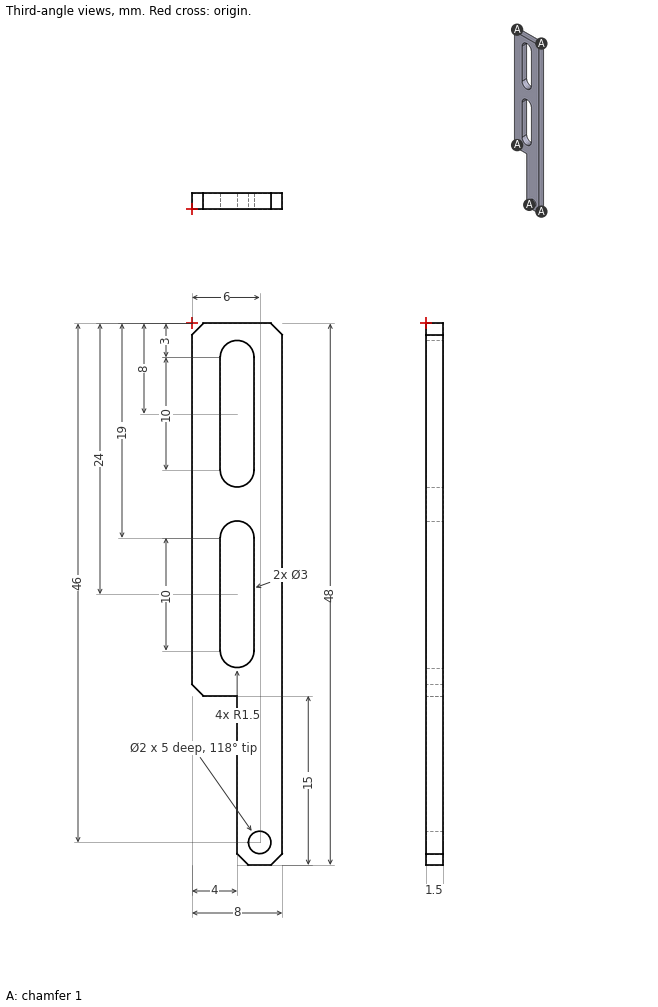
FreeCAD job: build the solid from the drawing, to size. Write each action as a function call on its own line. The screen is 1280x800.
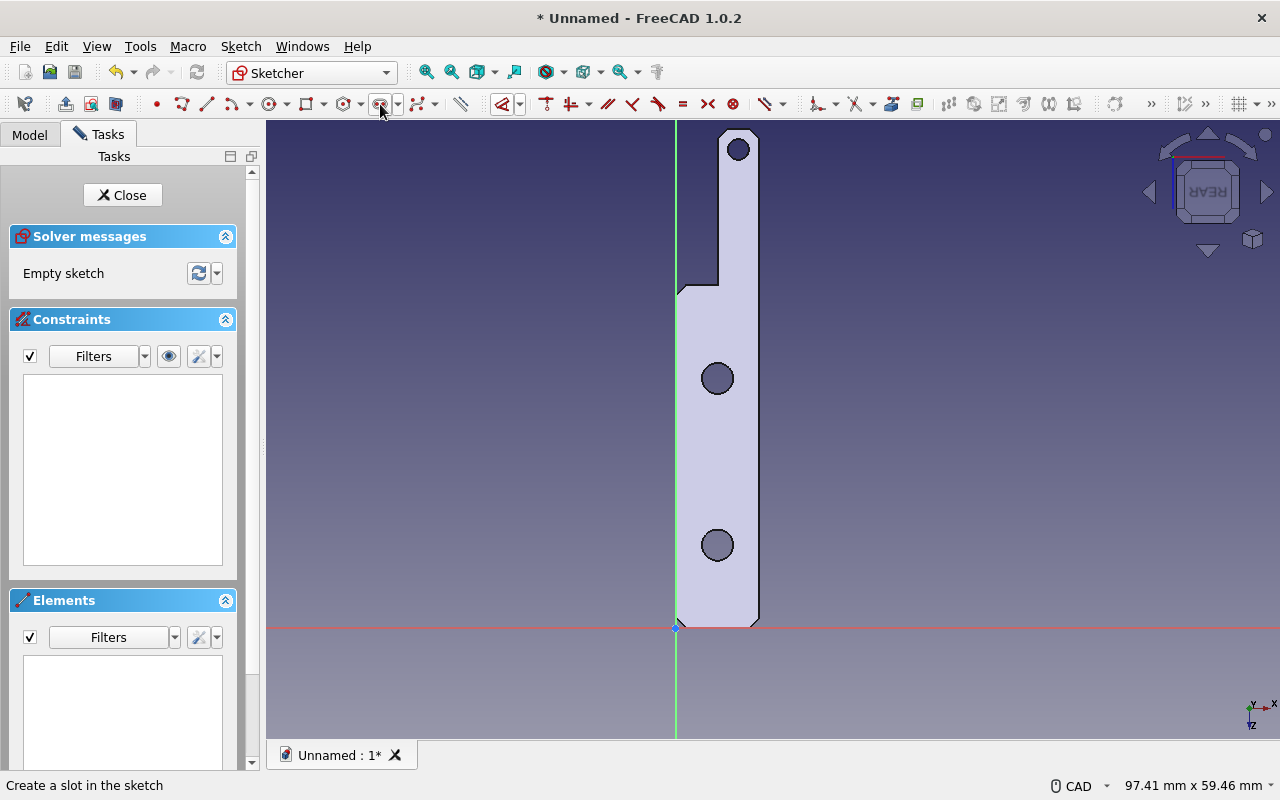
scroll(718, 431, up, 2)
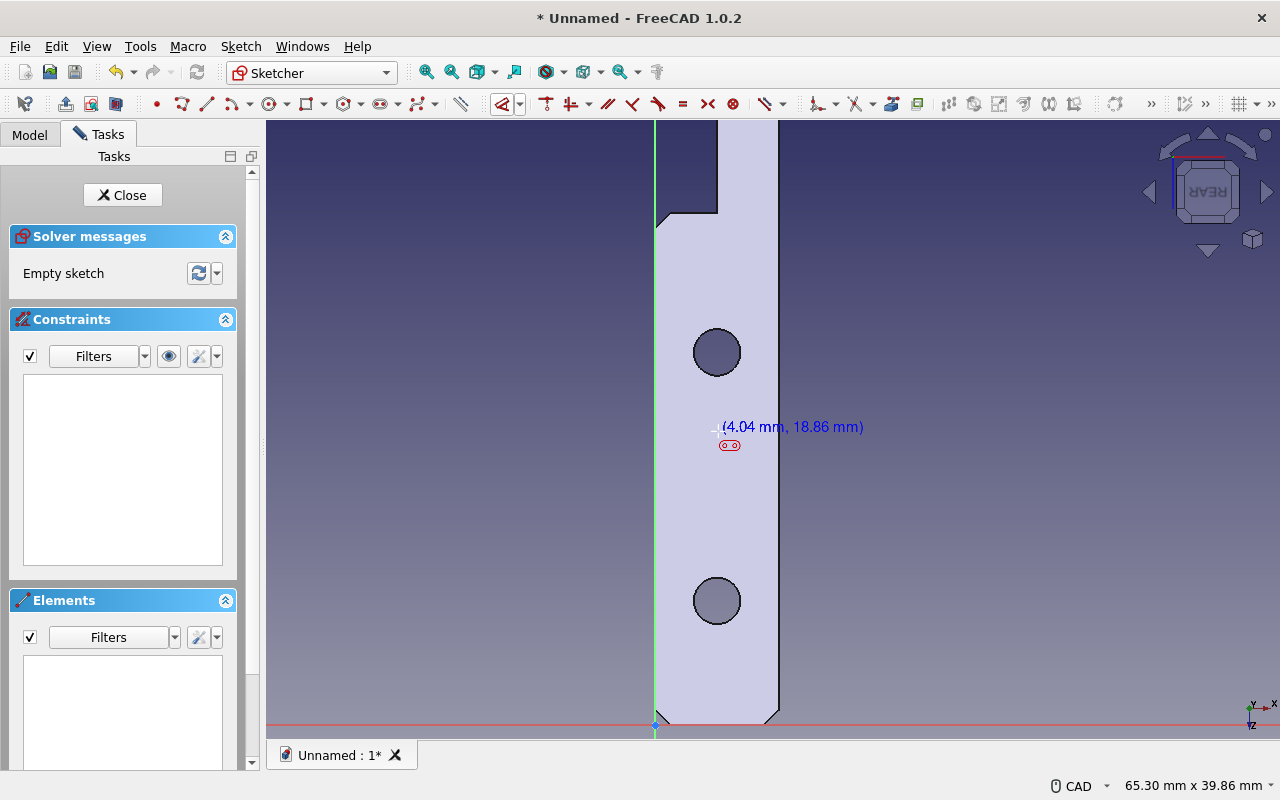
click(717, 430)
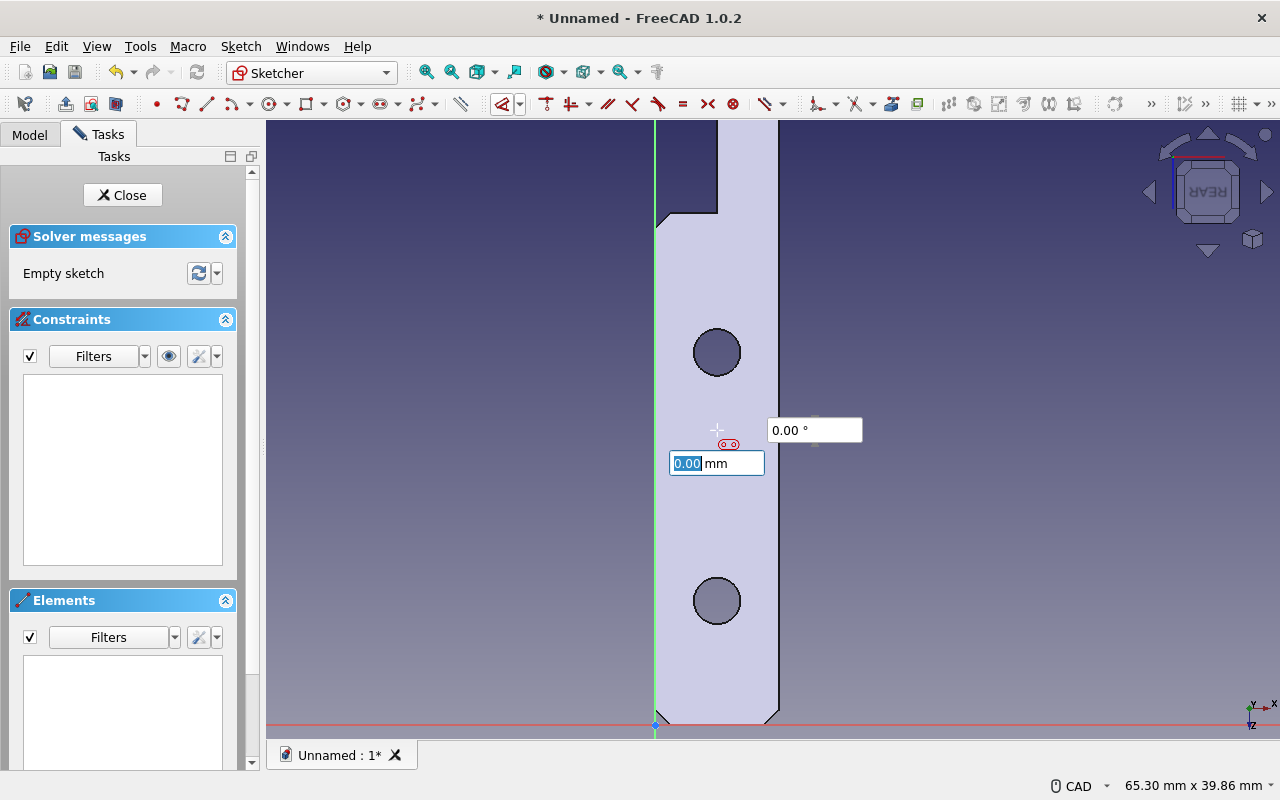
click(717, 275)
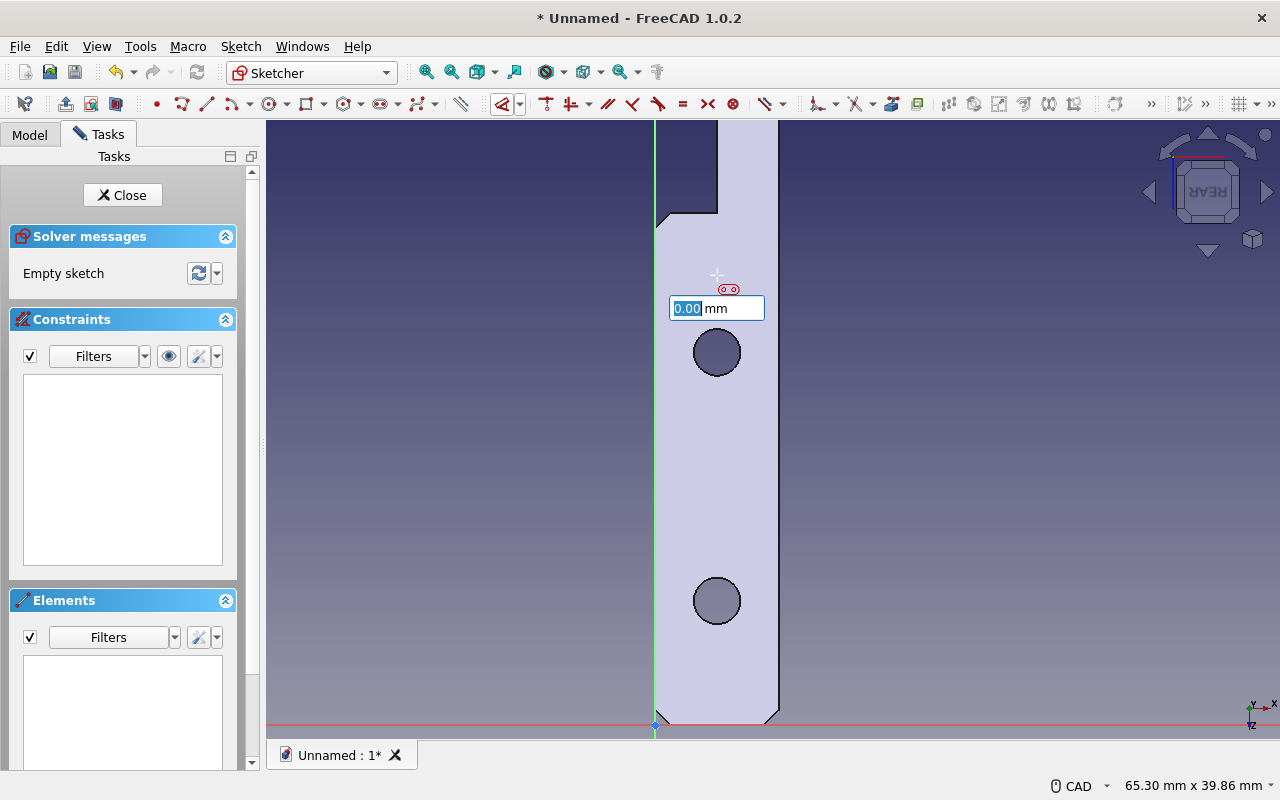
click(740, 352)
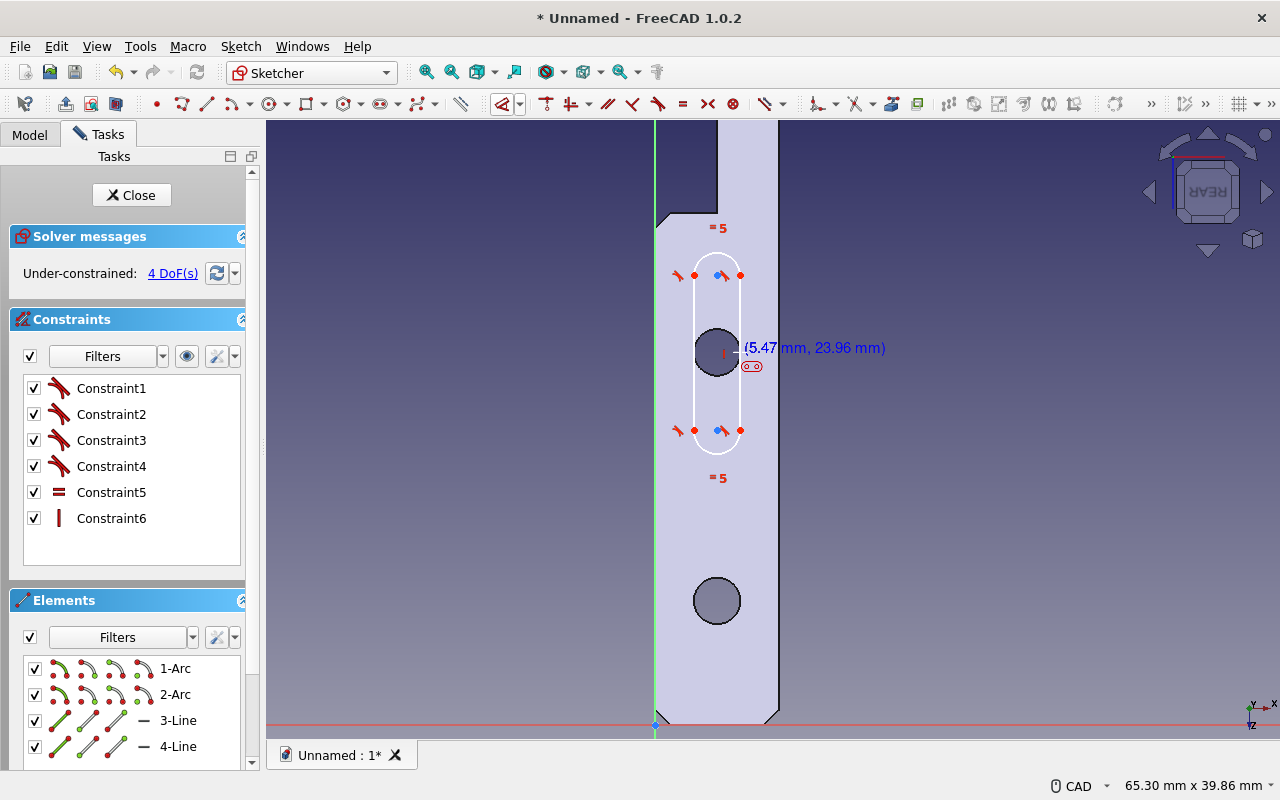
click(717, 679)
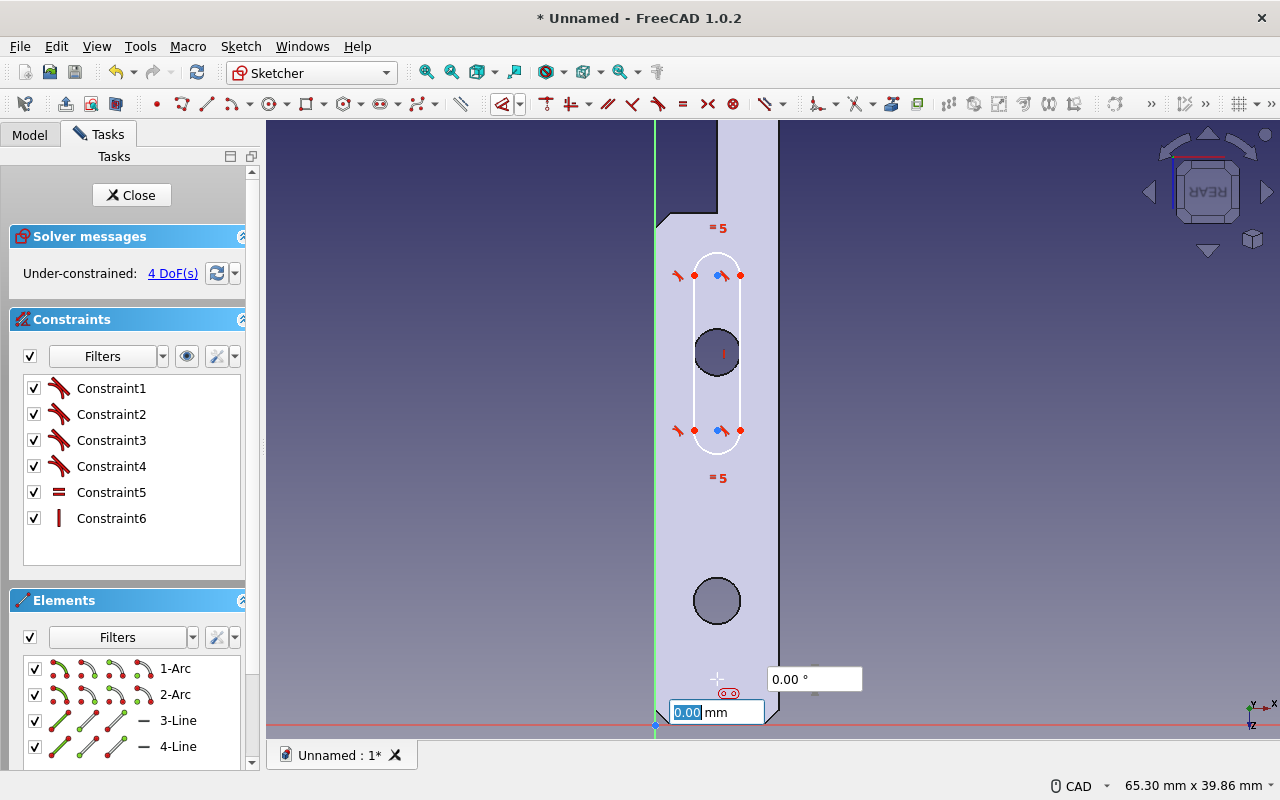
click(717, 523)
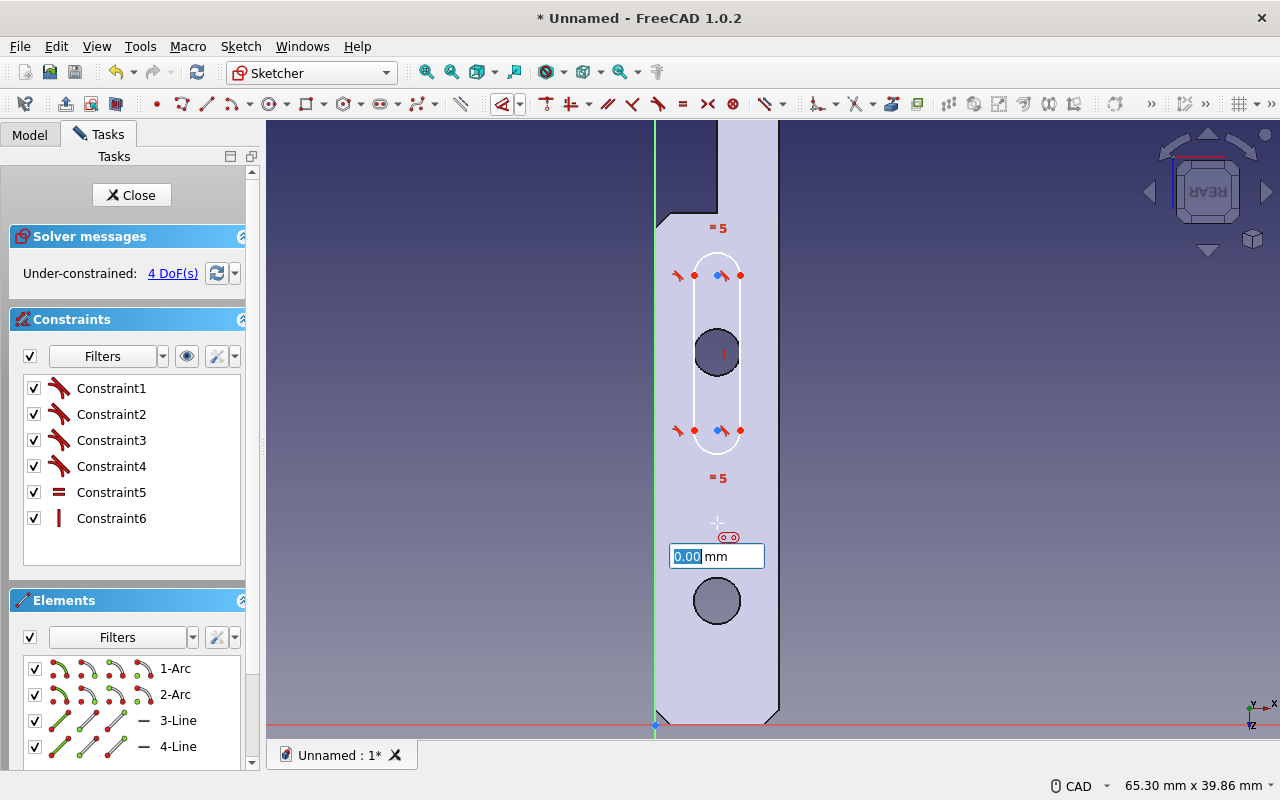
click(694, 601)
key(Escape)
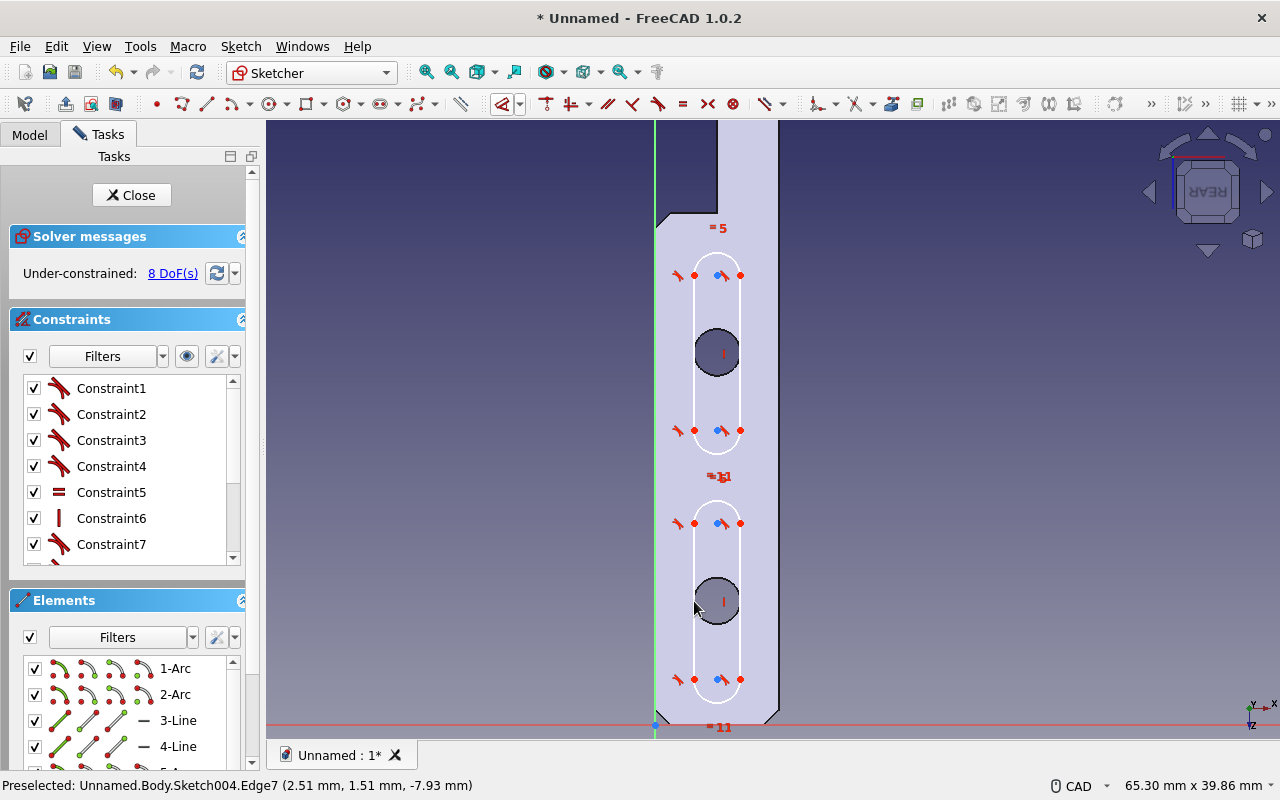
click(703, 450)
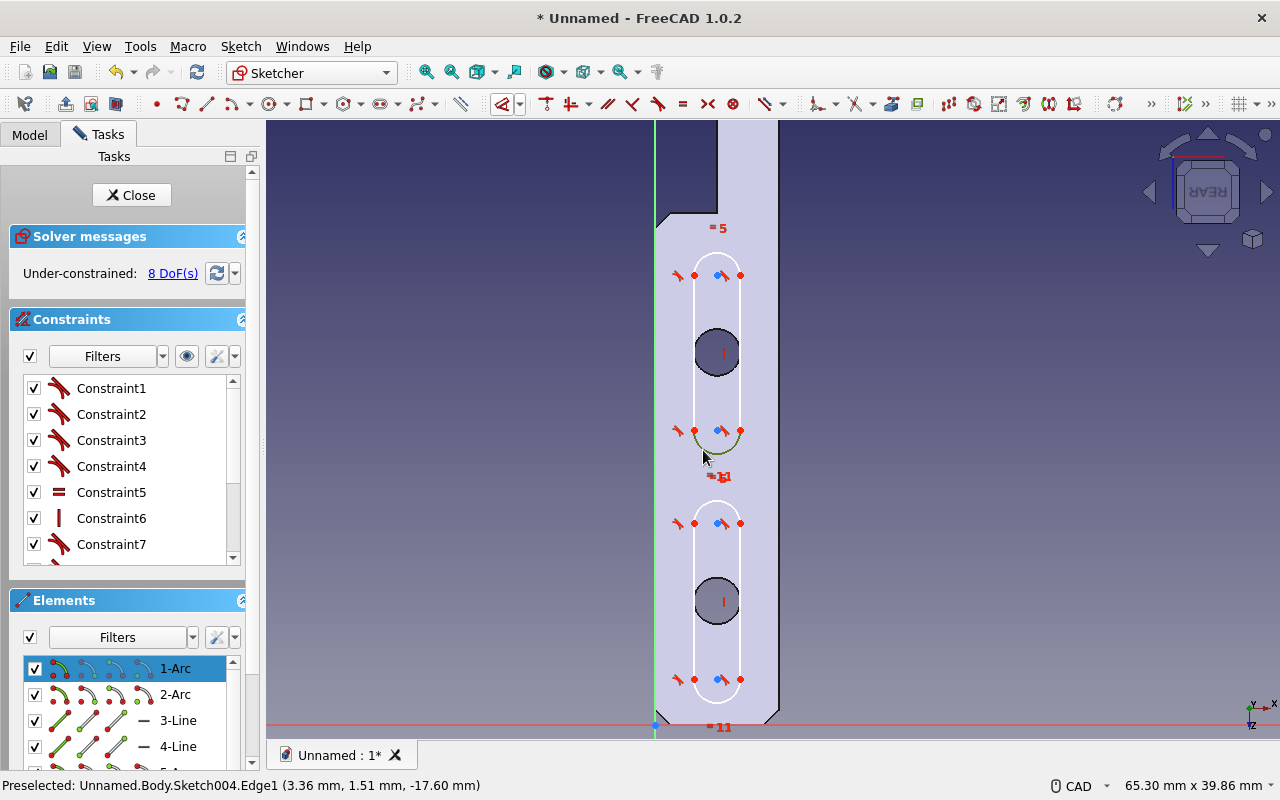
click(703, 699)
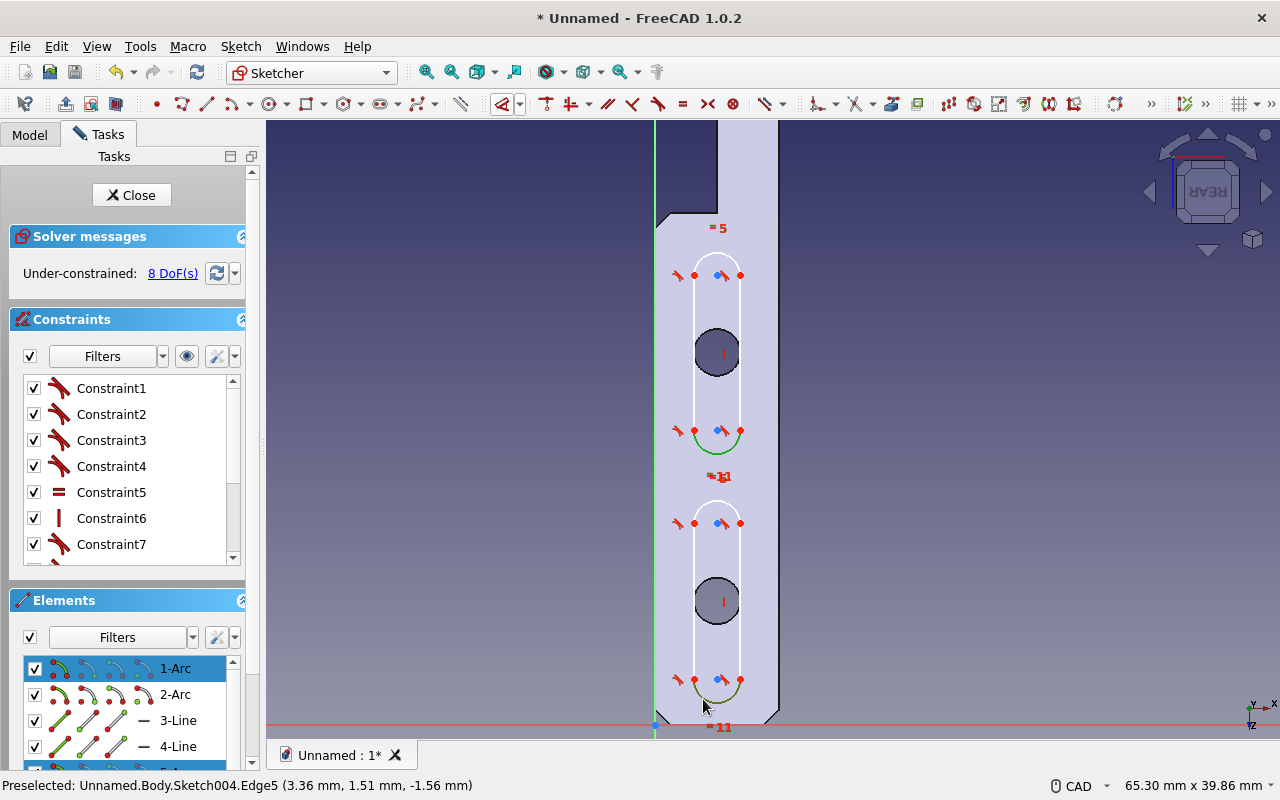
key(e)